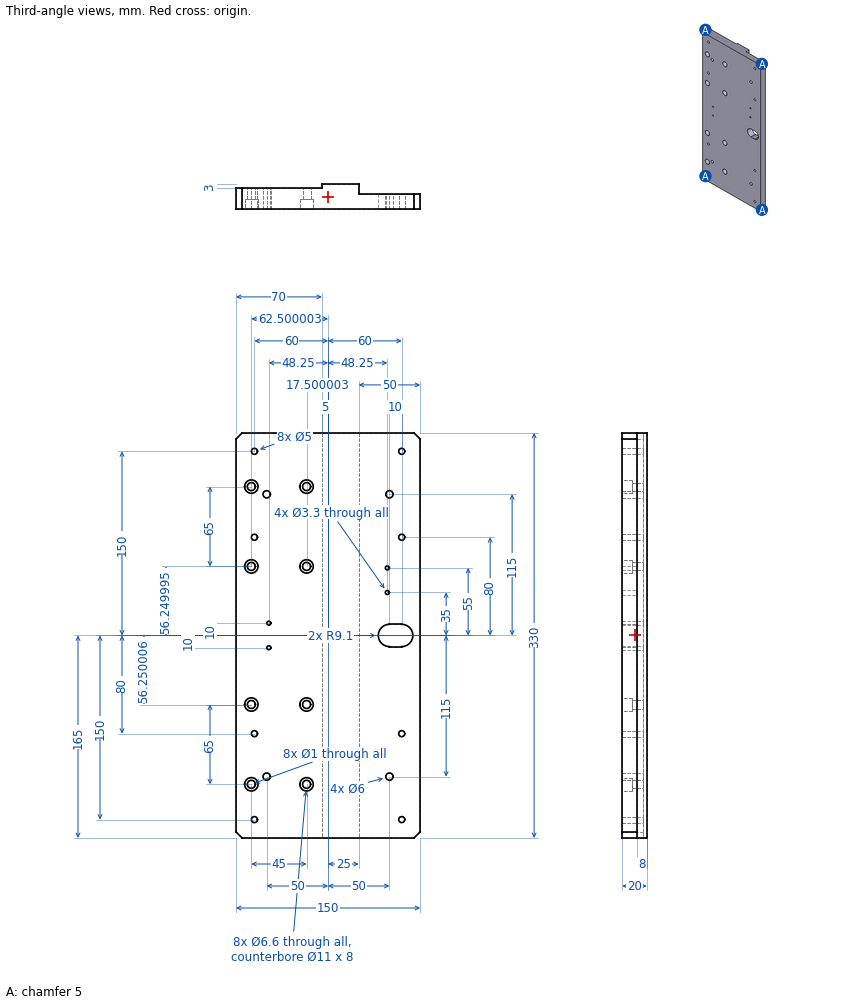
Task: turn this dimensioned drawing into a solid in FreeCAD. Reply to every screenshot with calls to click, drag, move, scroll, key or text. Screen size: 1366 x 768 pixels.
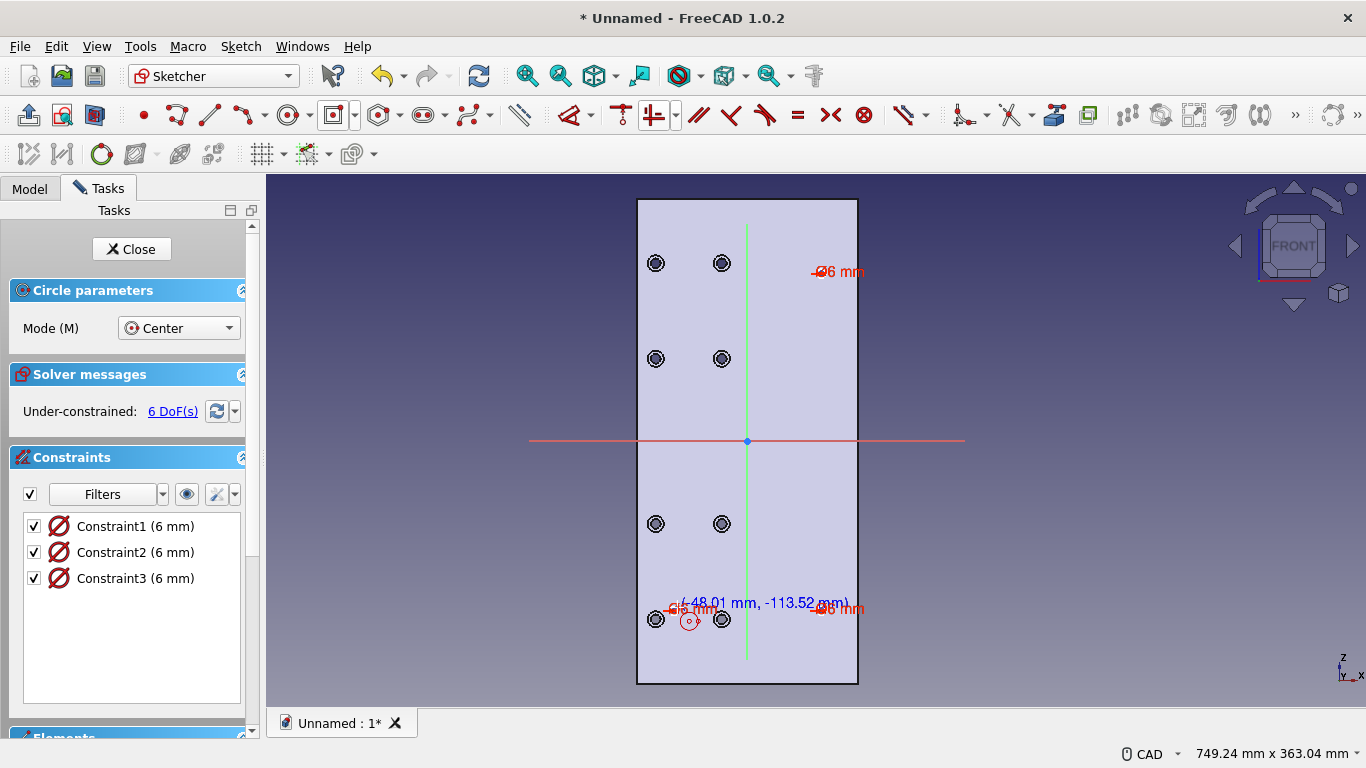
scroll(674, 272, up, 9)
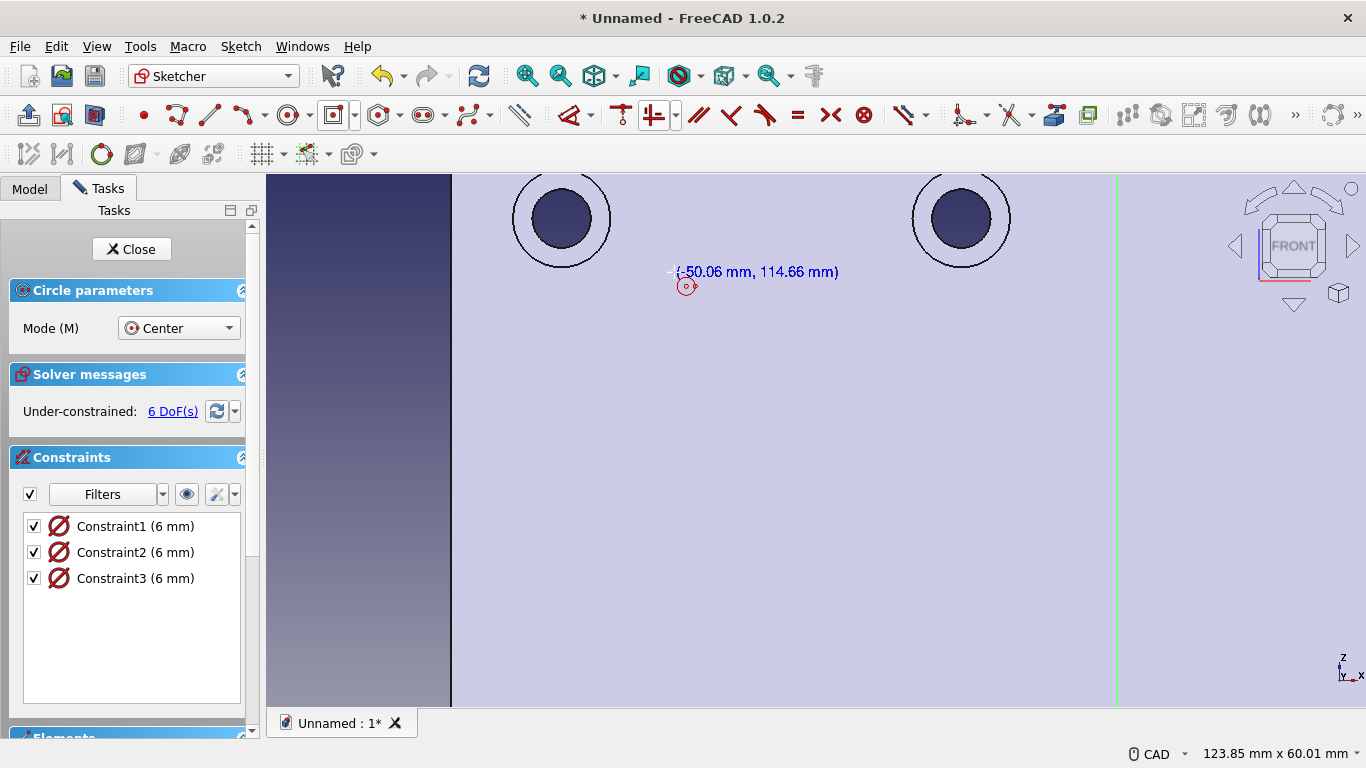
scroll(674, 271, down, 9)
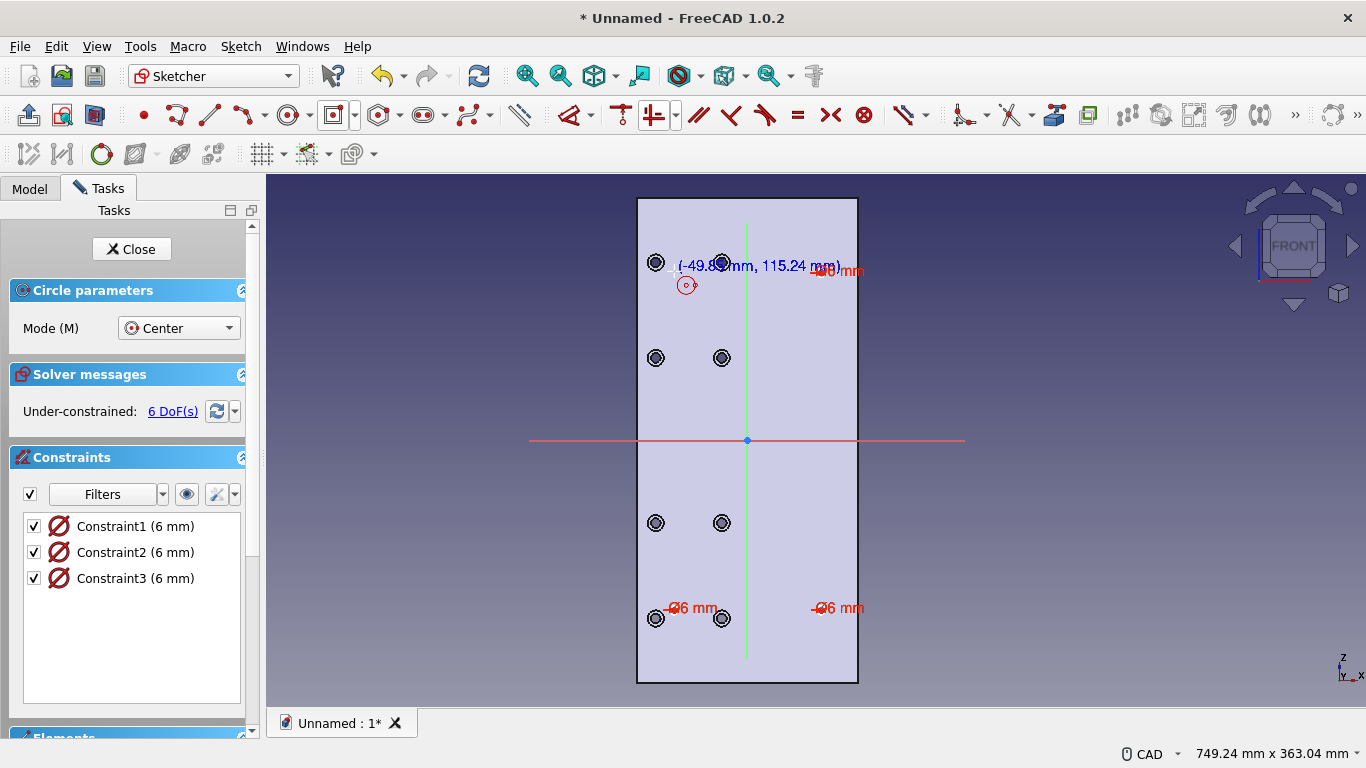
click(674, 272)
move(677, 269)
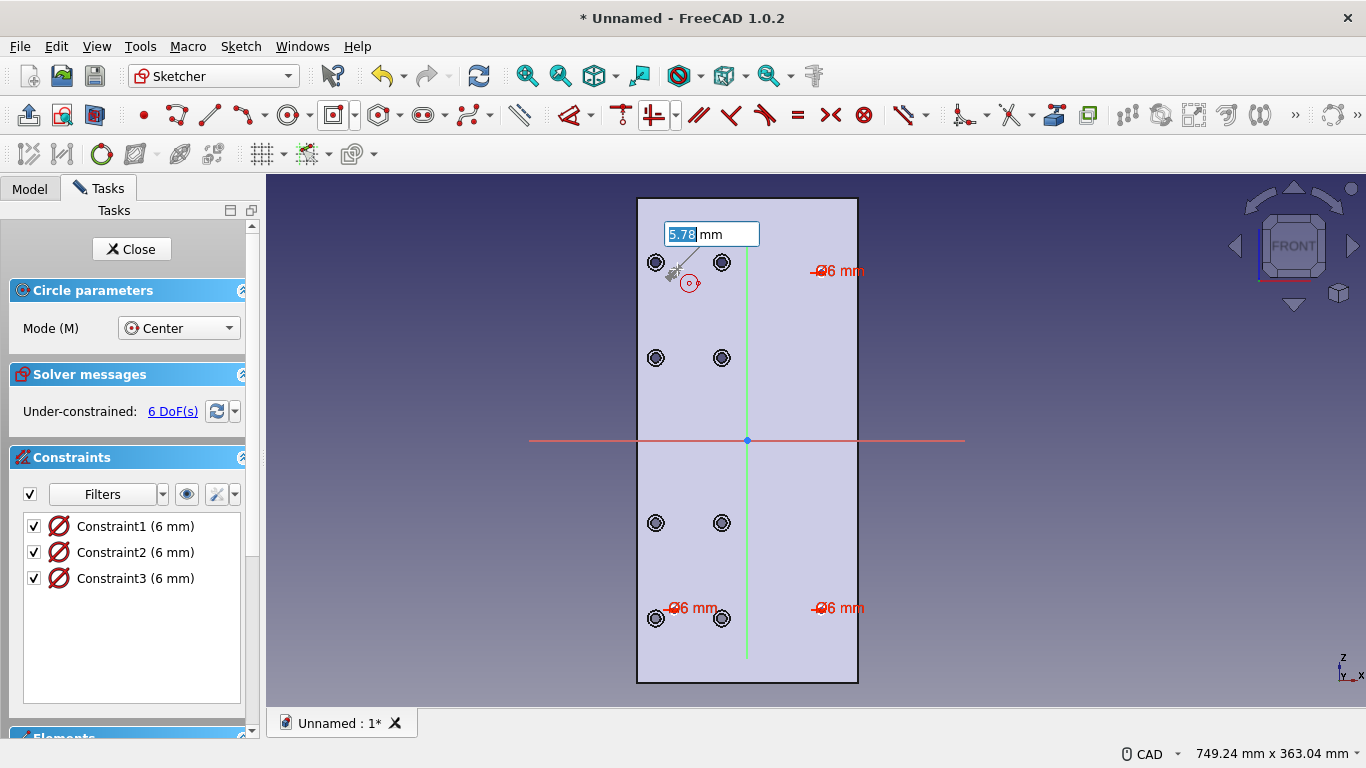
text(6)
key(Return)
key(Escape)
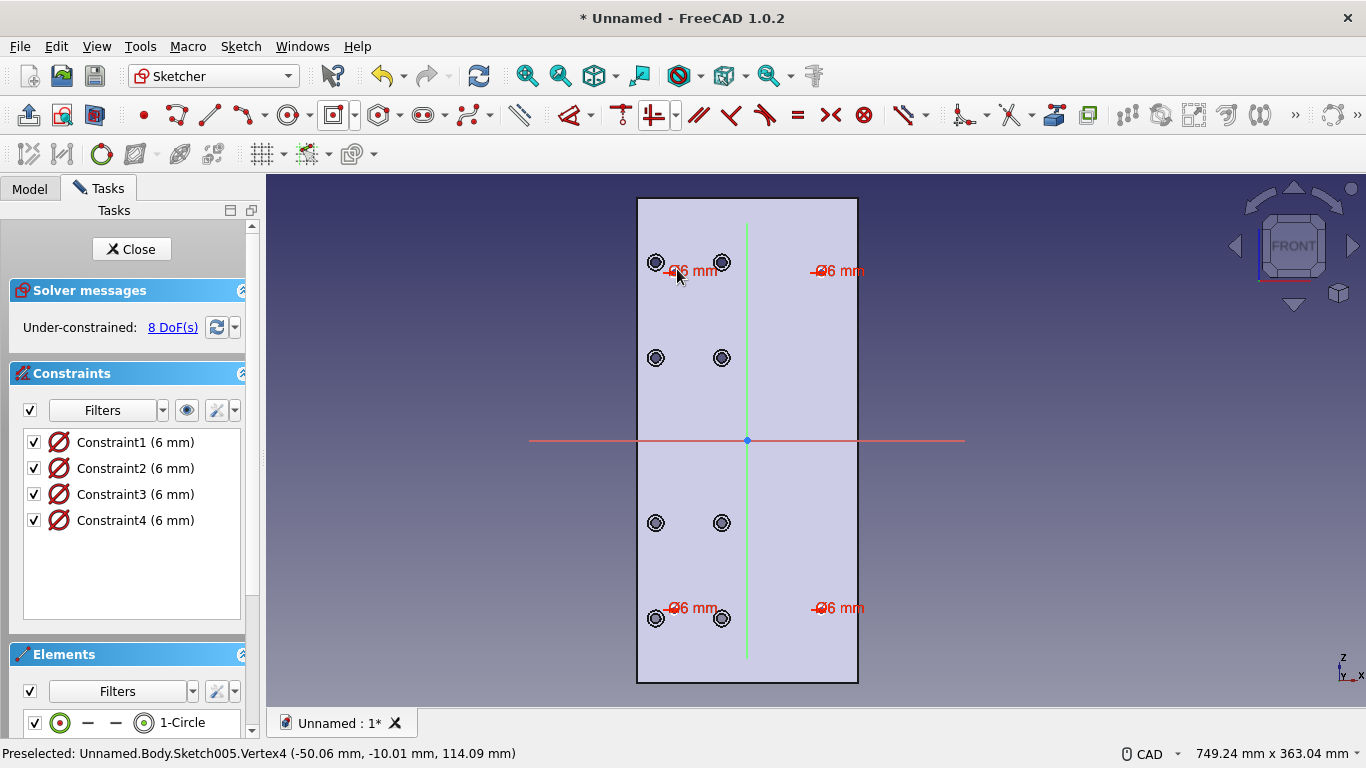
click(821, 610)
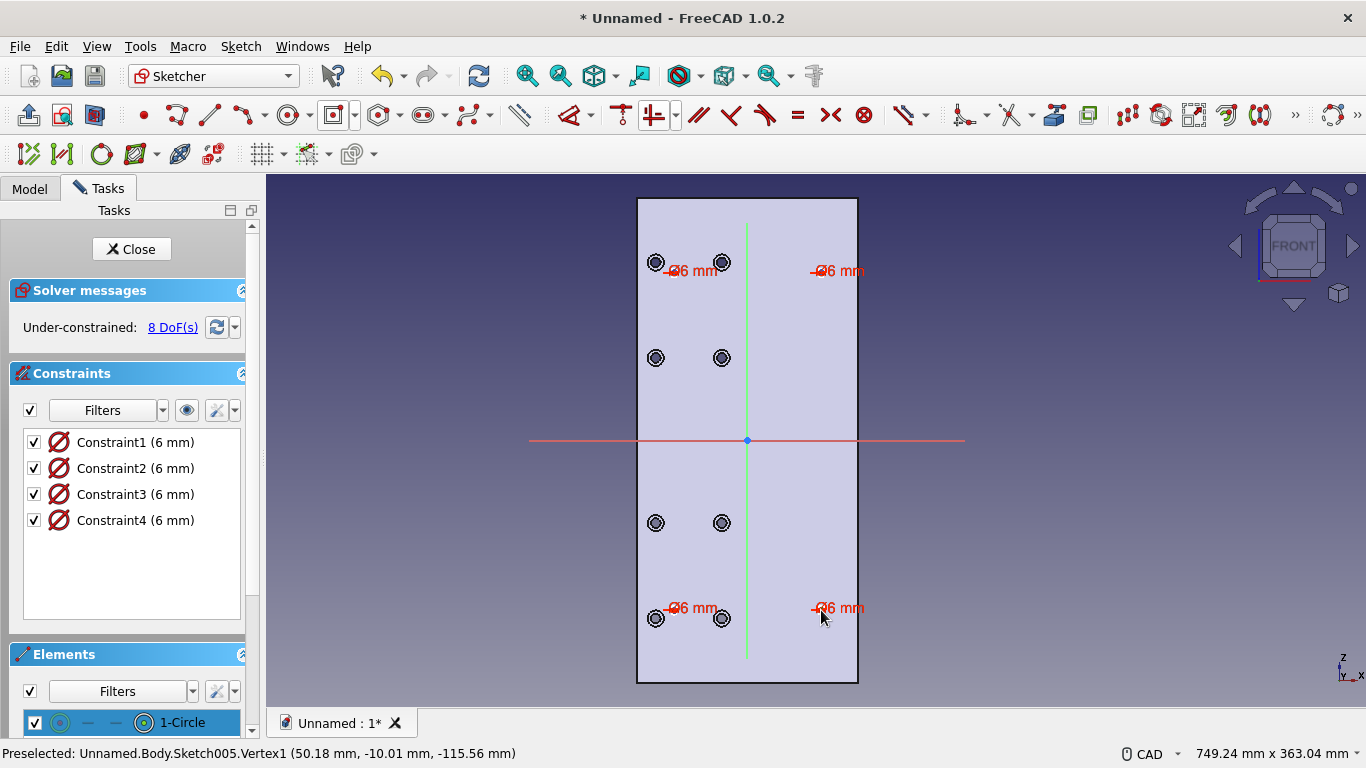
click(821, 273)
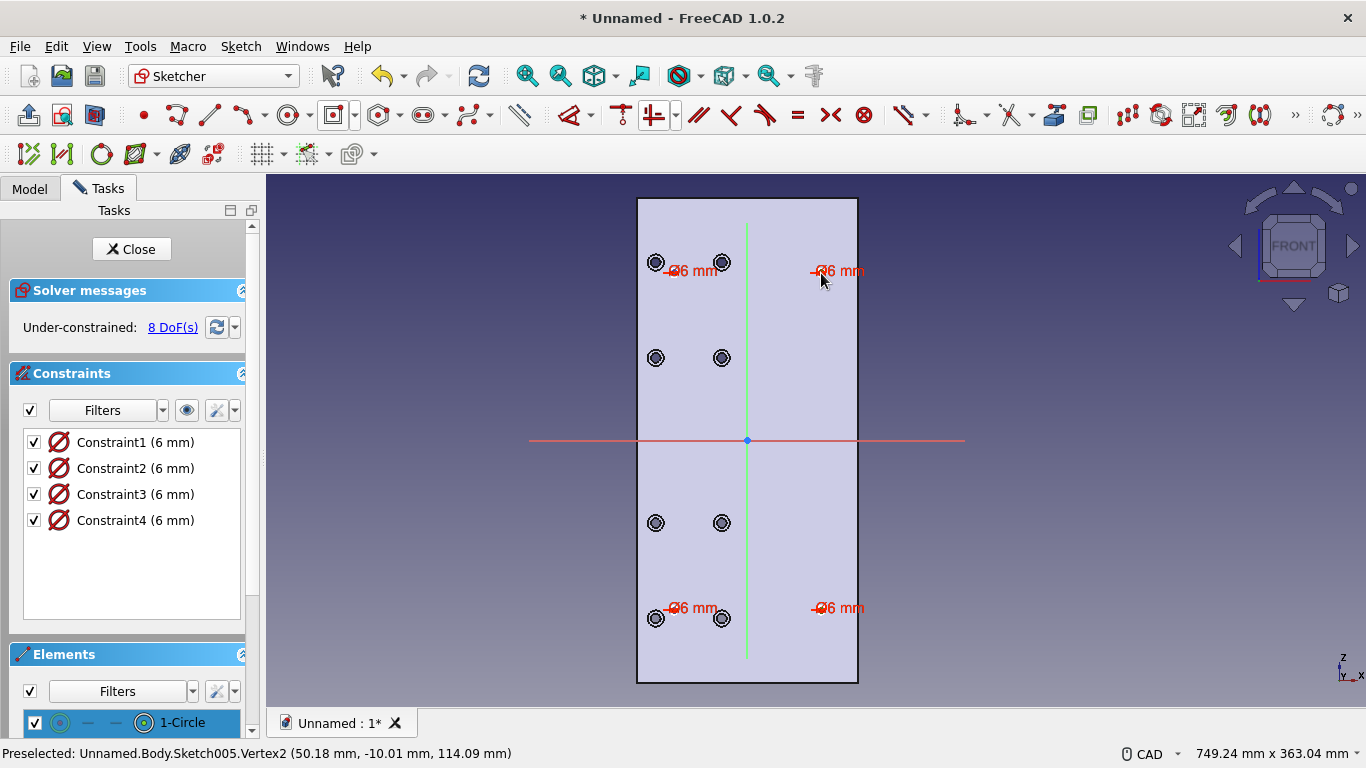
click(676, 116)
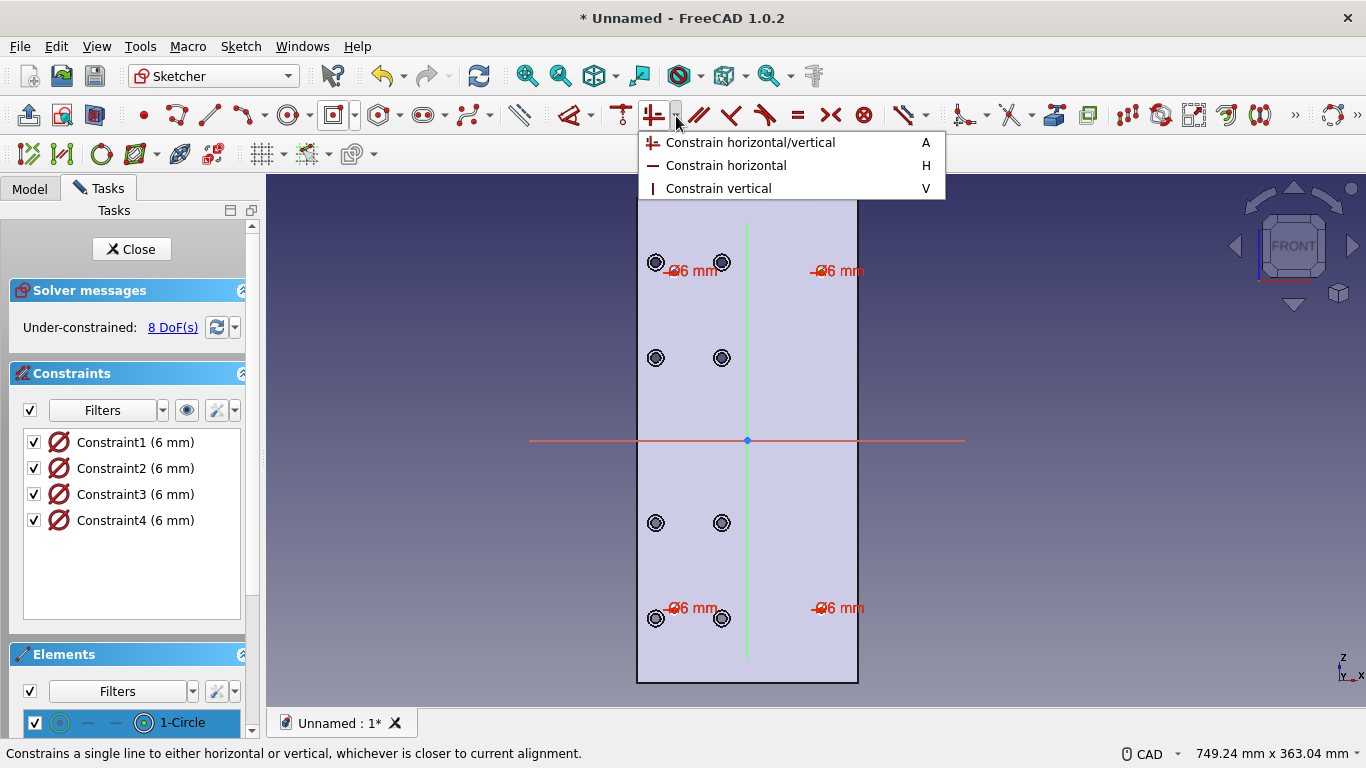
click(792, 188)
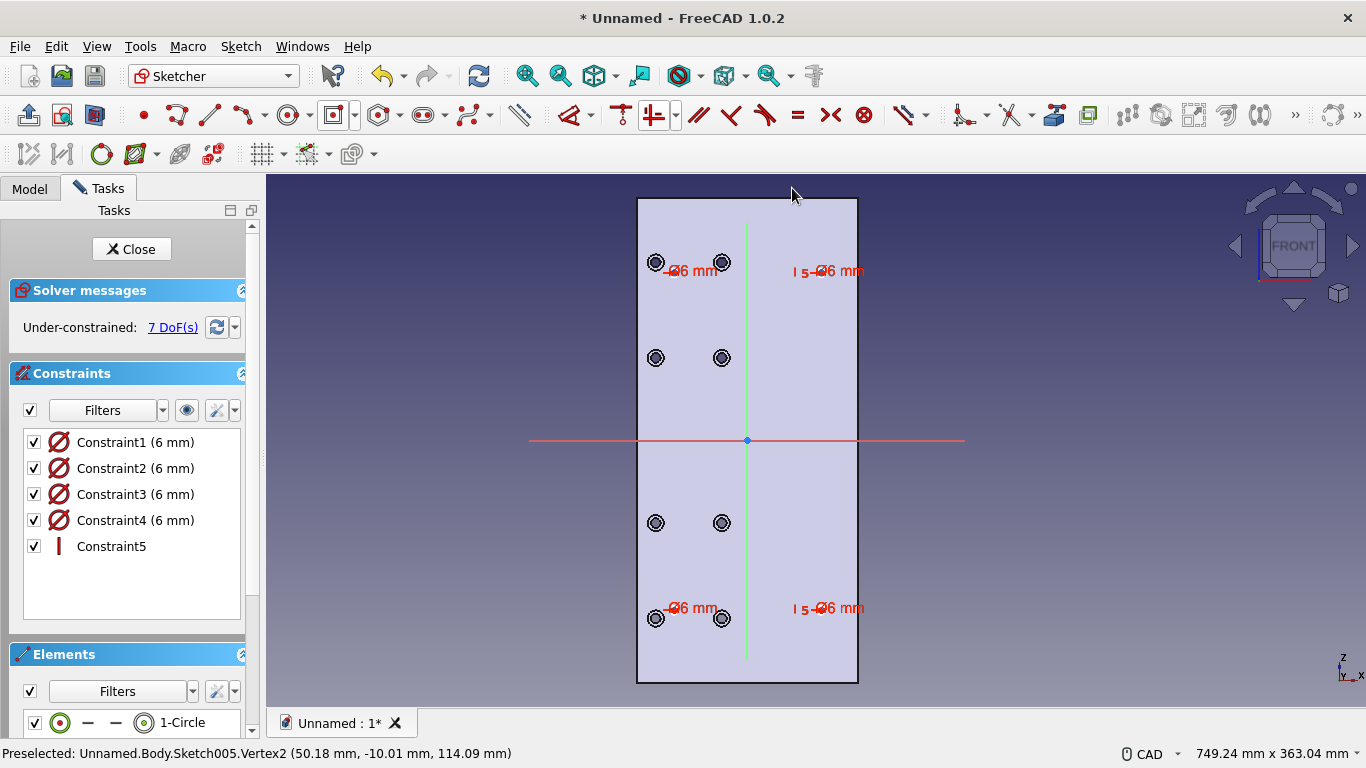
click(821, 610)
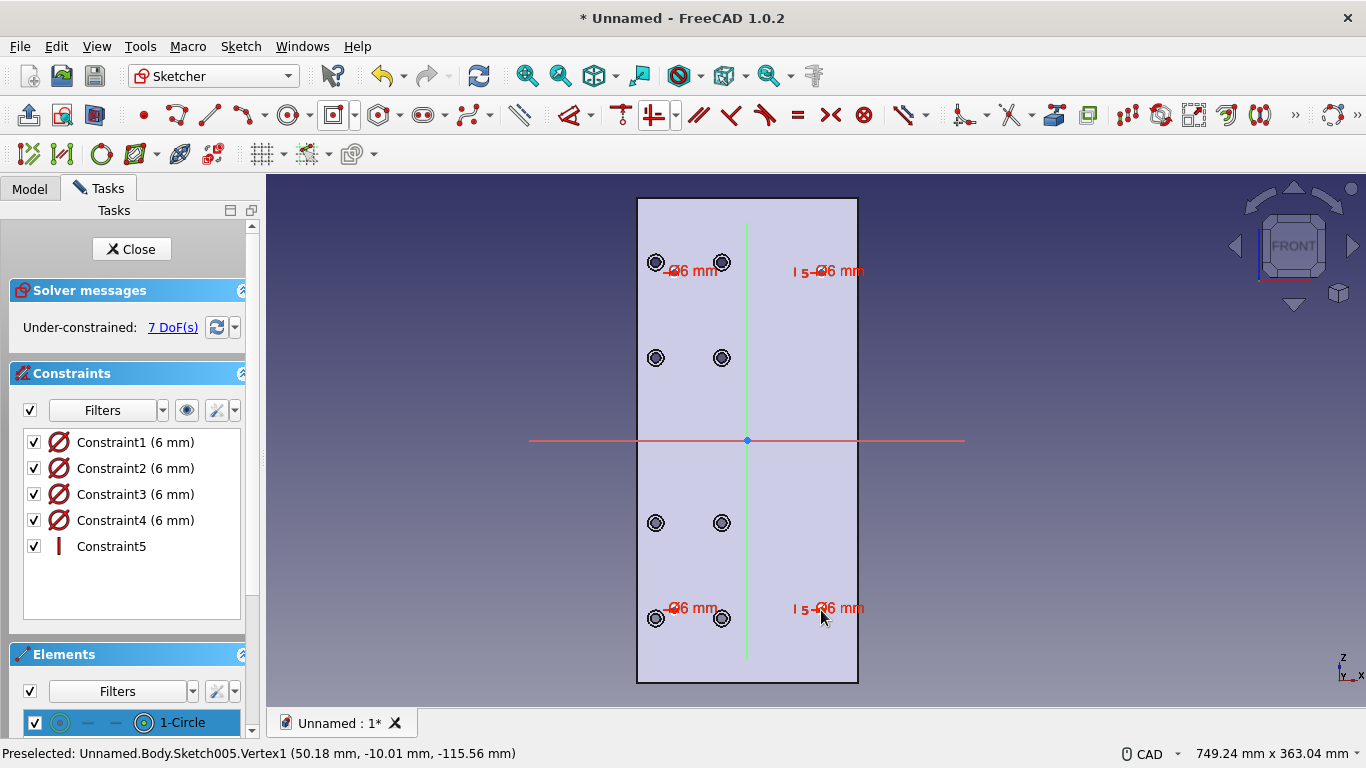
click(674, 610)